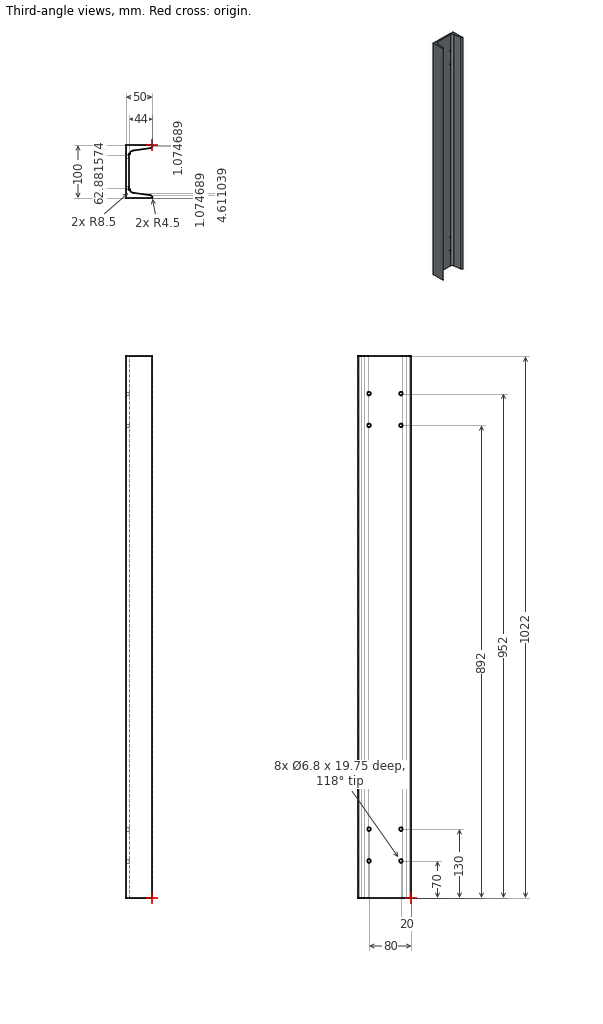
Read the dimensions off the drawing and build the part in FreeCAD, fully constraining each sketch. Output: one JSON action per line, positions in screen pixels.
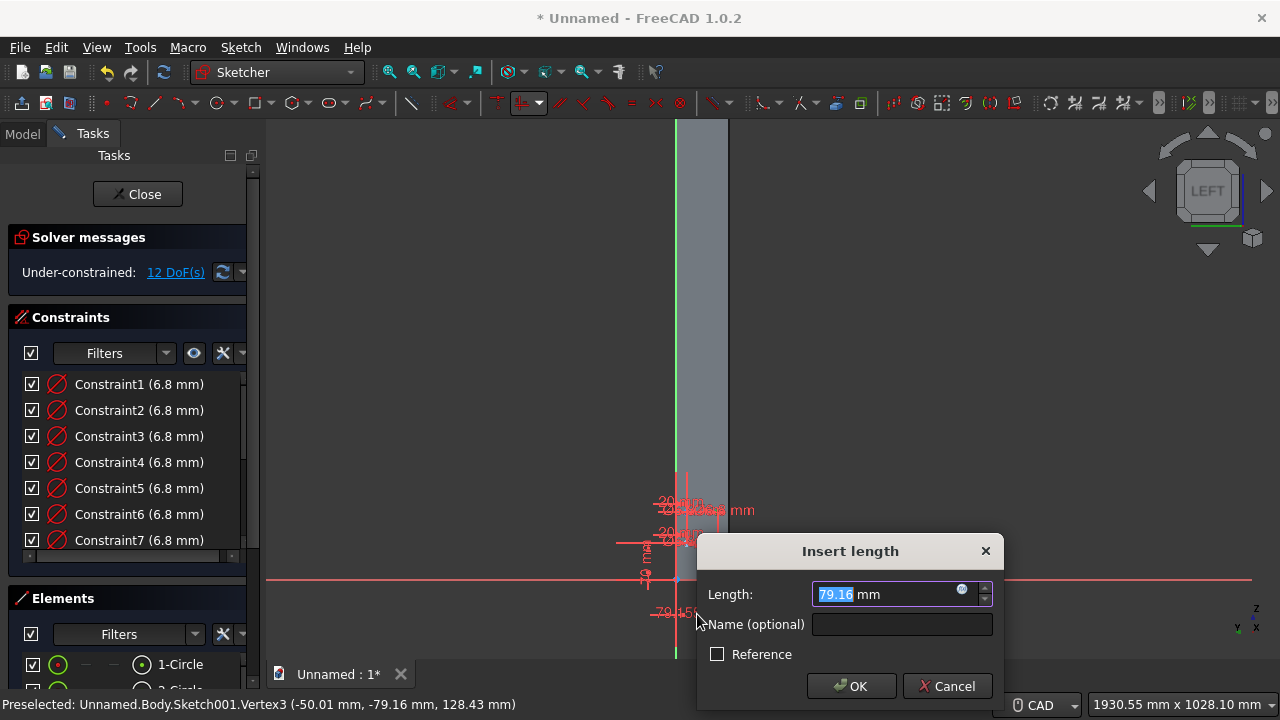
{"action": "type", "text": "80"}
{"action": "key", "text": "Return"}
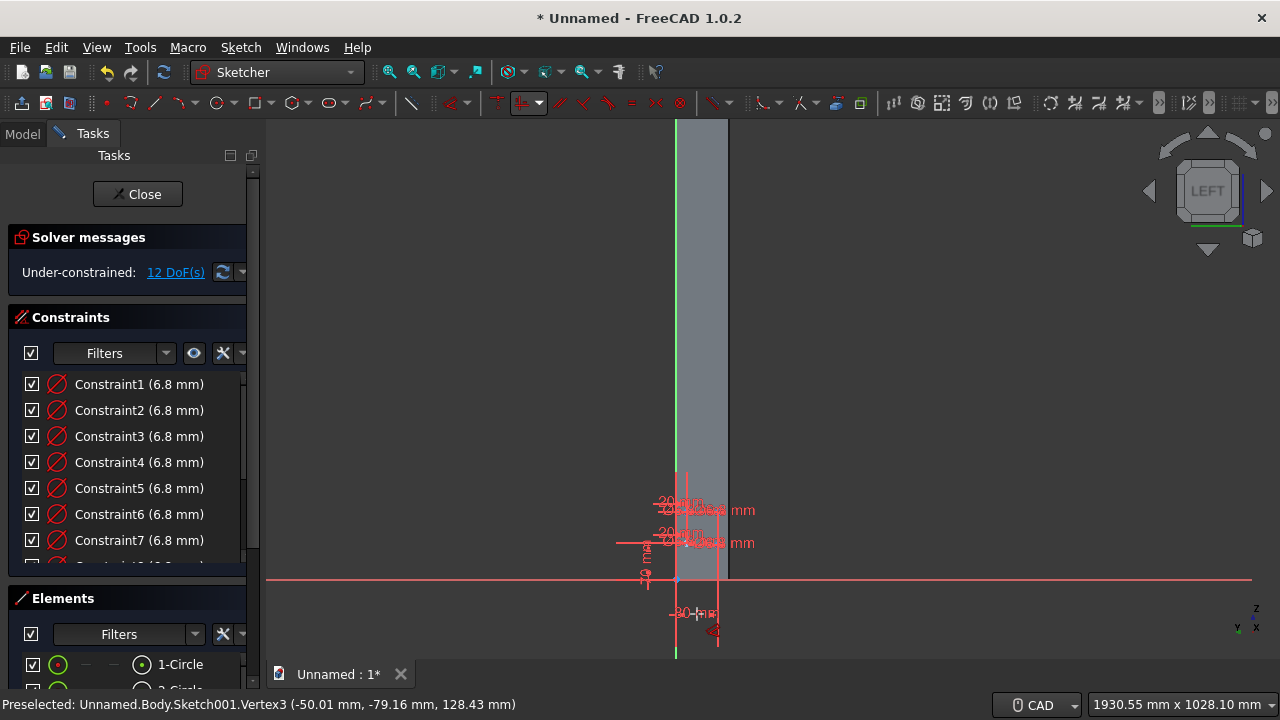
{"action": "left_click", "coordinate": [718, 545]}
{"action": "left_click", "coordinate": [697, 463]}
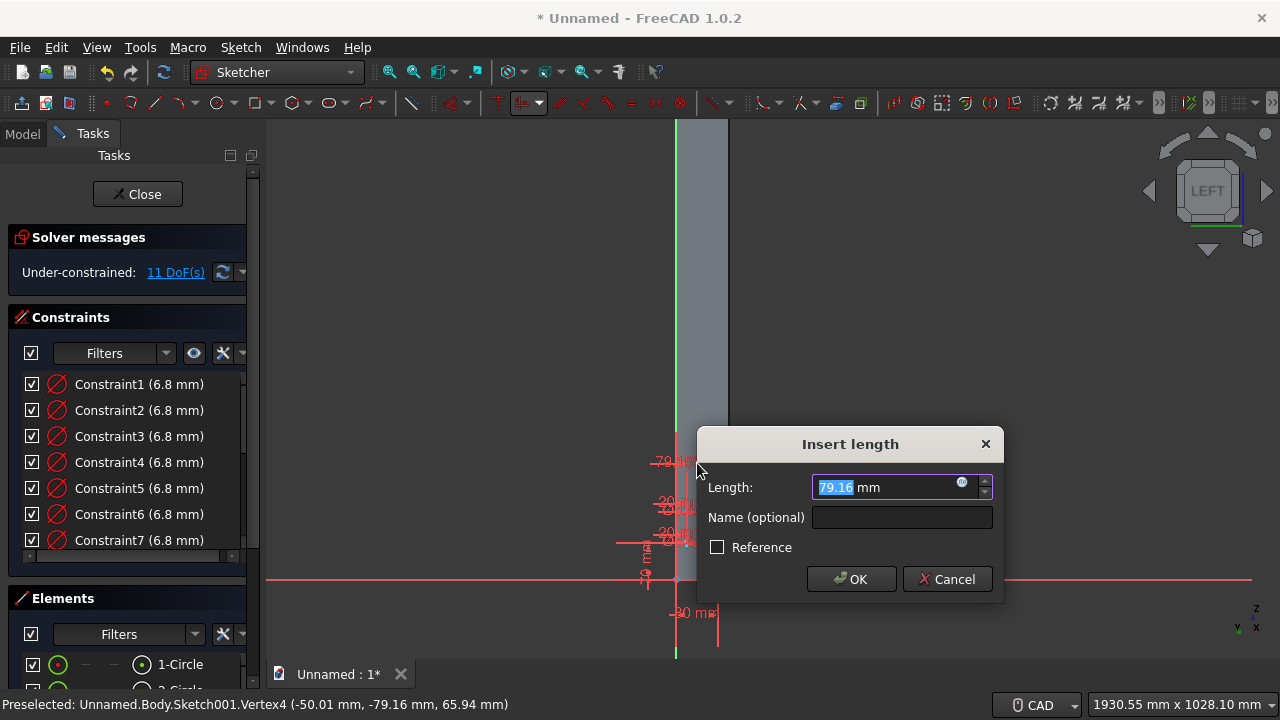
{"action": "type", "text": "80"}
{"action": "key", "text": "Return"}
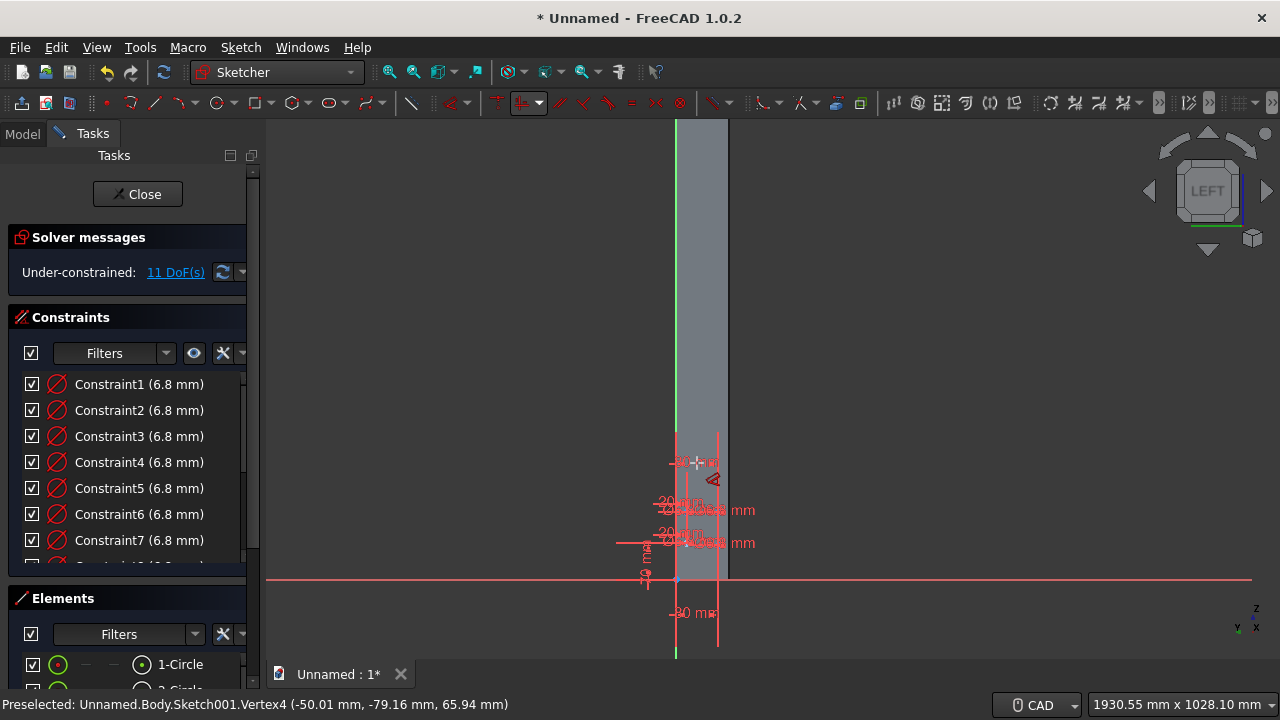
{"action": "left_click", "coordinate": [718, 545]}
{"action": "left_click", "coordinate": [752, 563]}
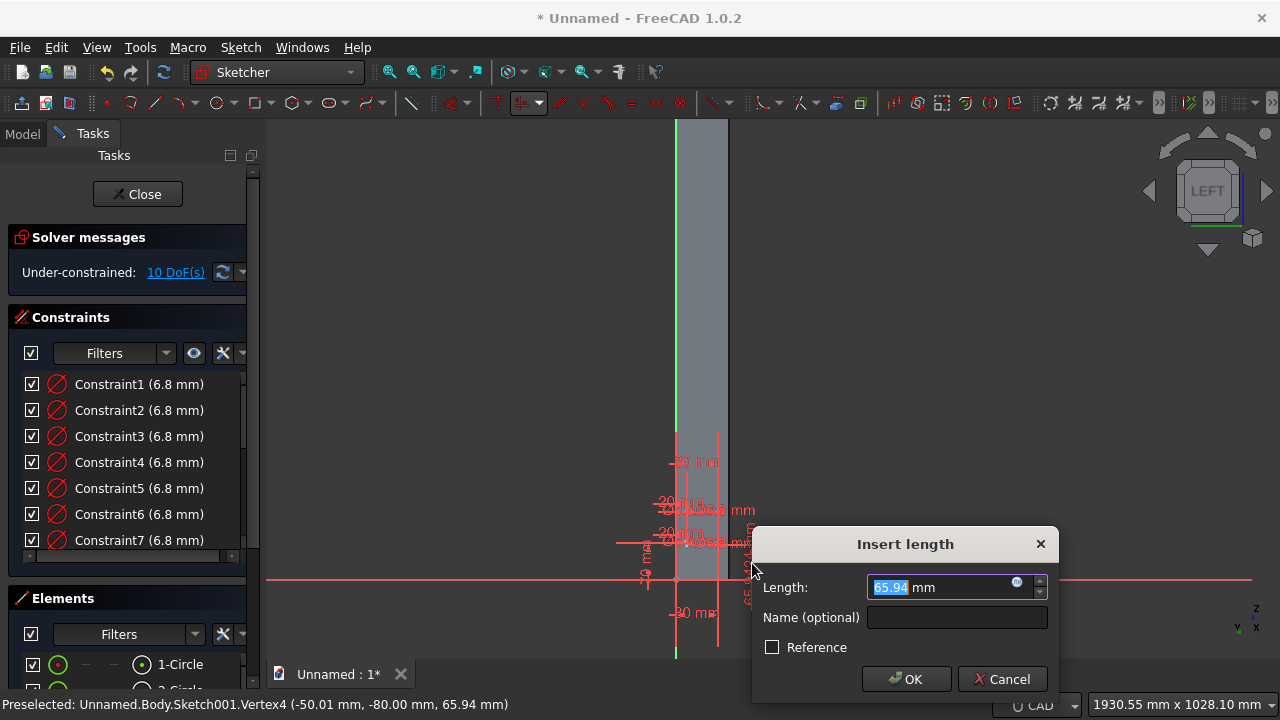
{"action": "type", "text": "70"}
{"action": "key", "text": "Return"}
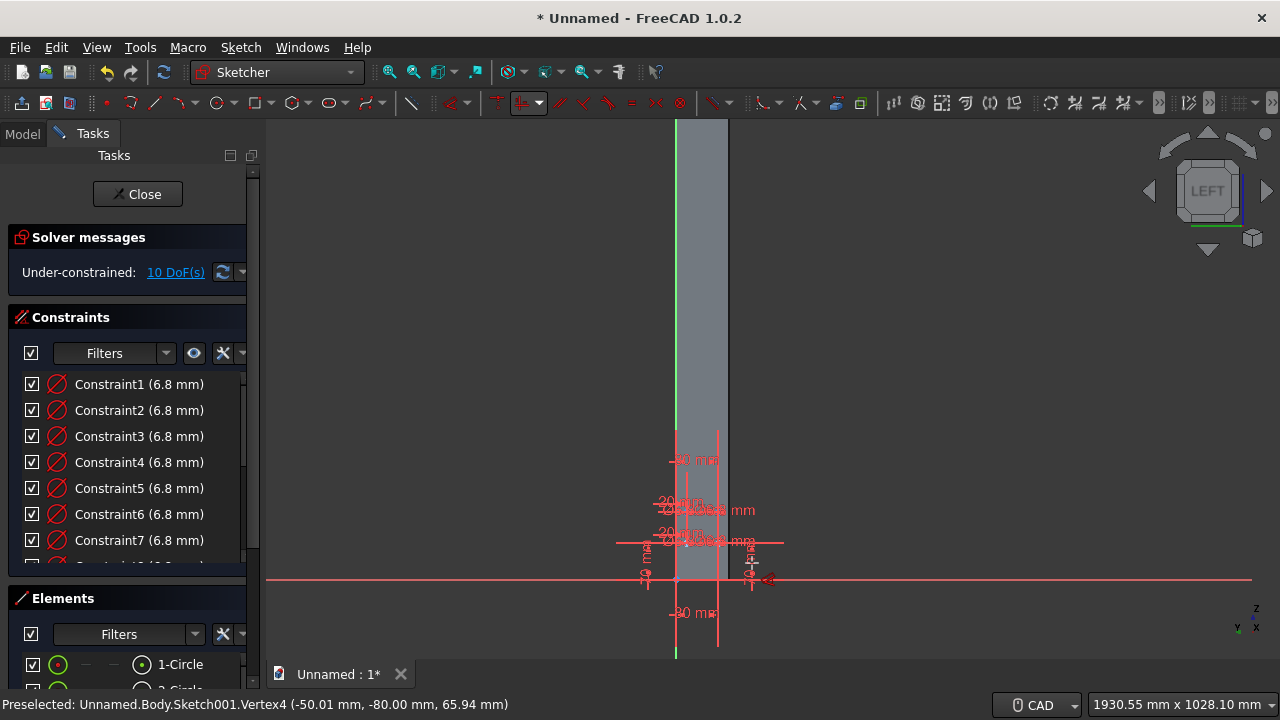
{"action": "scroll", "coordinate": [718, 511], "scroll_direction": "down", "scroll_amount": 2}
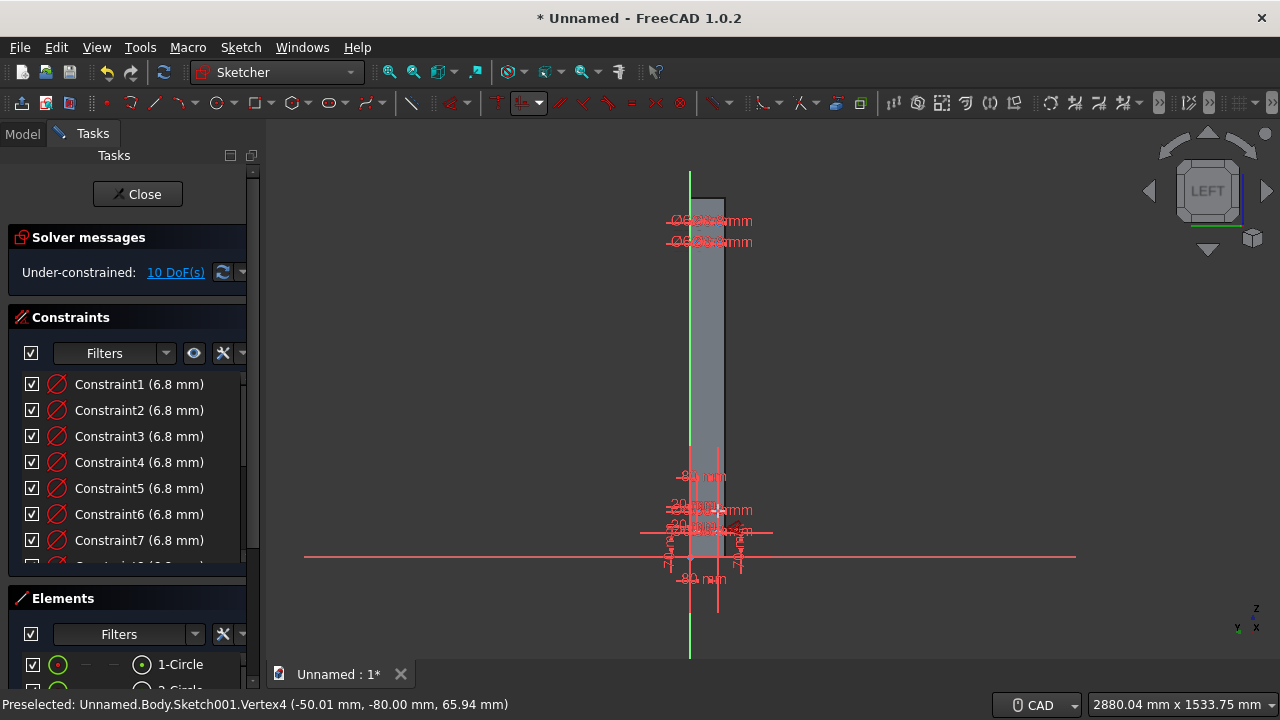
{"action": "scroll", "coordinate": [697, 244], "scroll_direction": "up", "scroll_amount": 9}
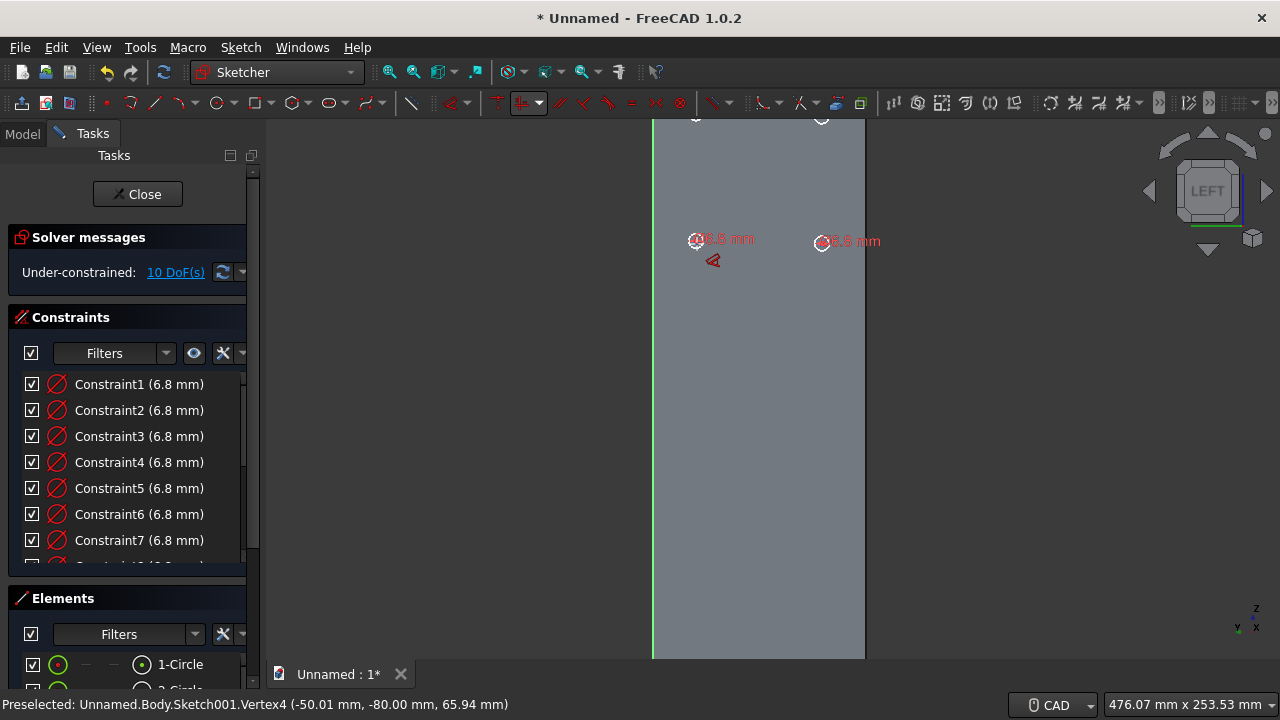
{"action": "left_click", "coordinate": [696, 241]}
{"action": "left_click", "coordinate": [674, 207]}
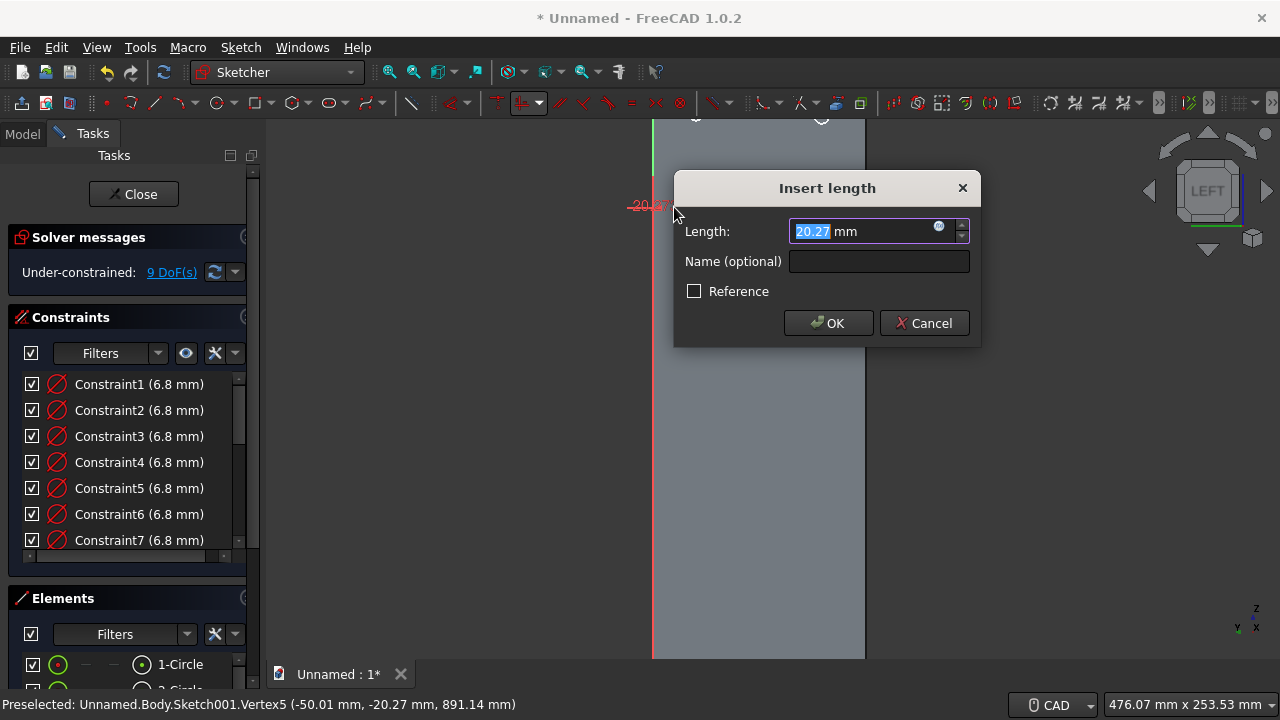
{"action": "type", "text": "20"}
{"action": "key", "text": "Return"}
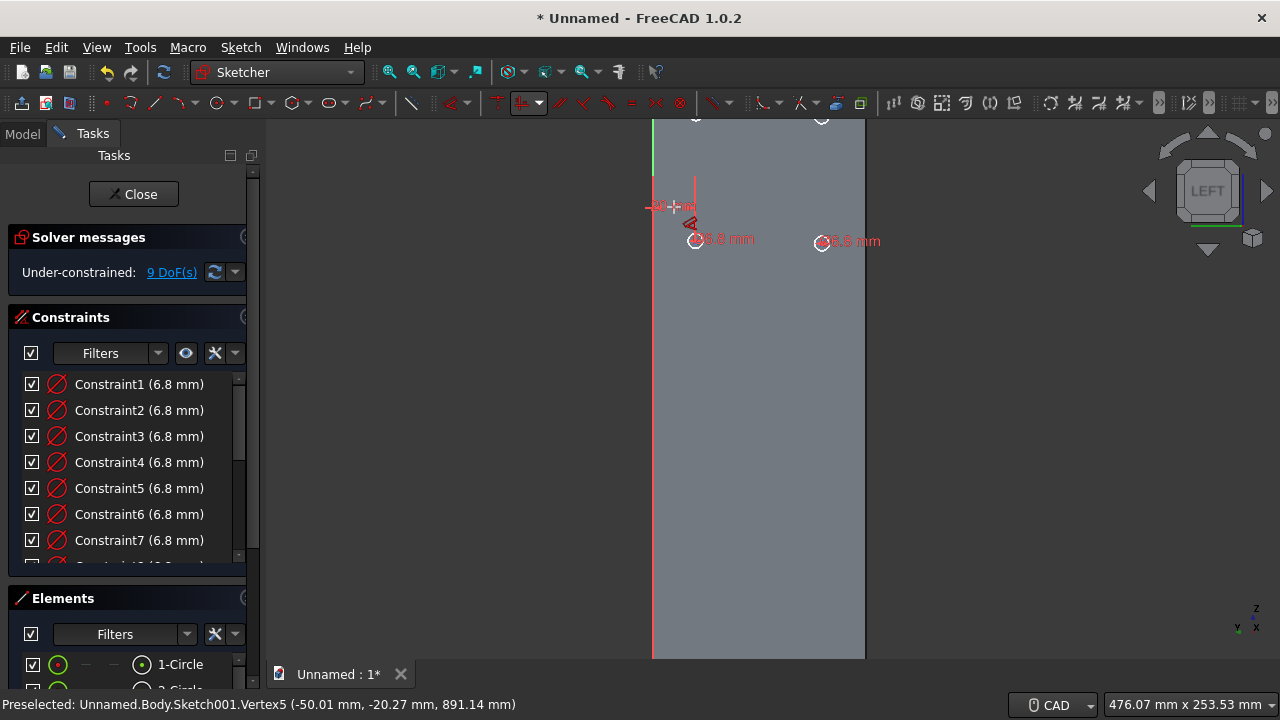
{"action": "scroll", "coordinate": [697, 244], "scroll_direction": "down", "scroll_amount": 9}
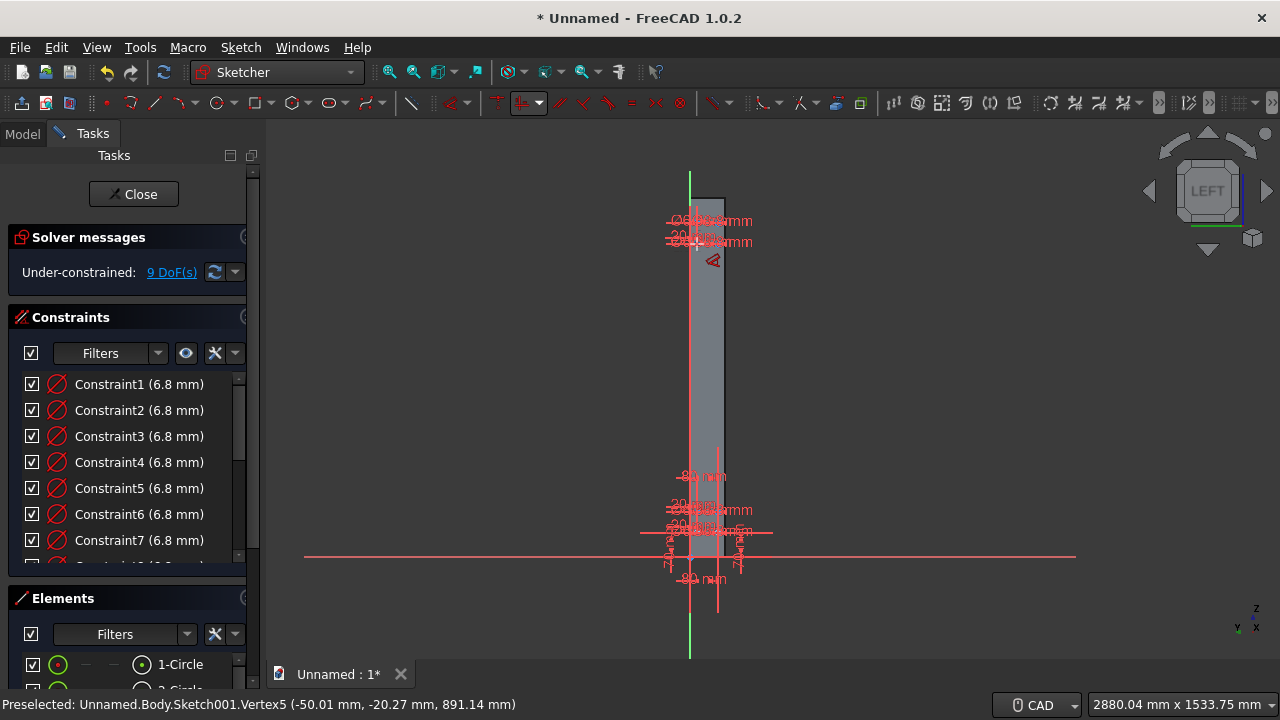
{"action": "scroll", "coordinate": [697, 223], "scroll_direction": "up", "scroll_amount": 9}